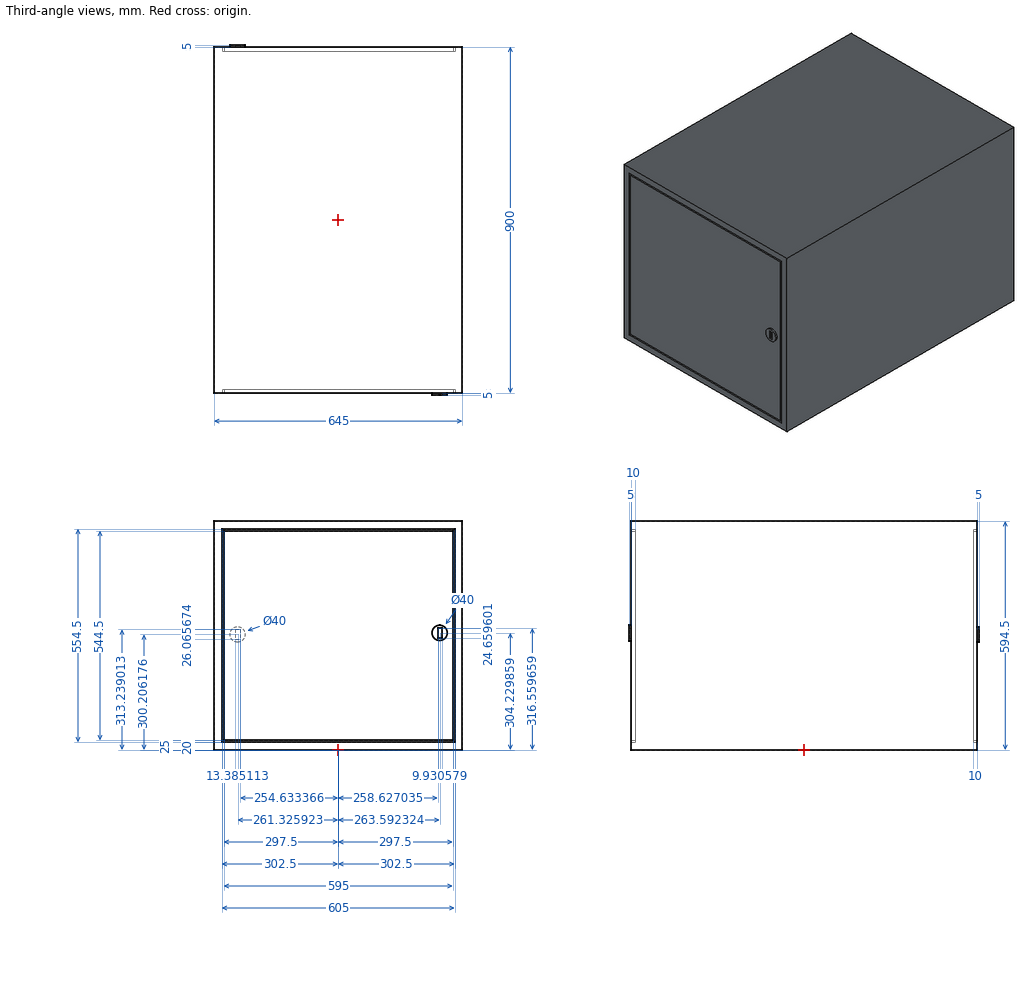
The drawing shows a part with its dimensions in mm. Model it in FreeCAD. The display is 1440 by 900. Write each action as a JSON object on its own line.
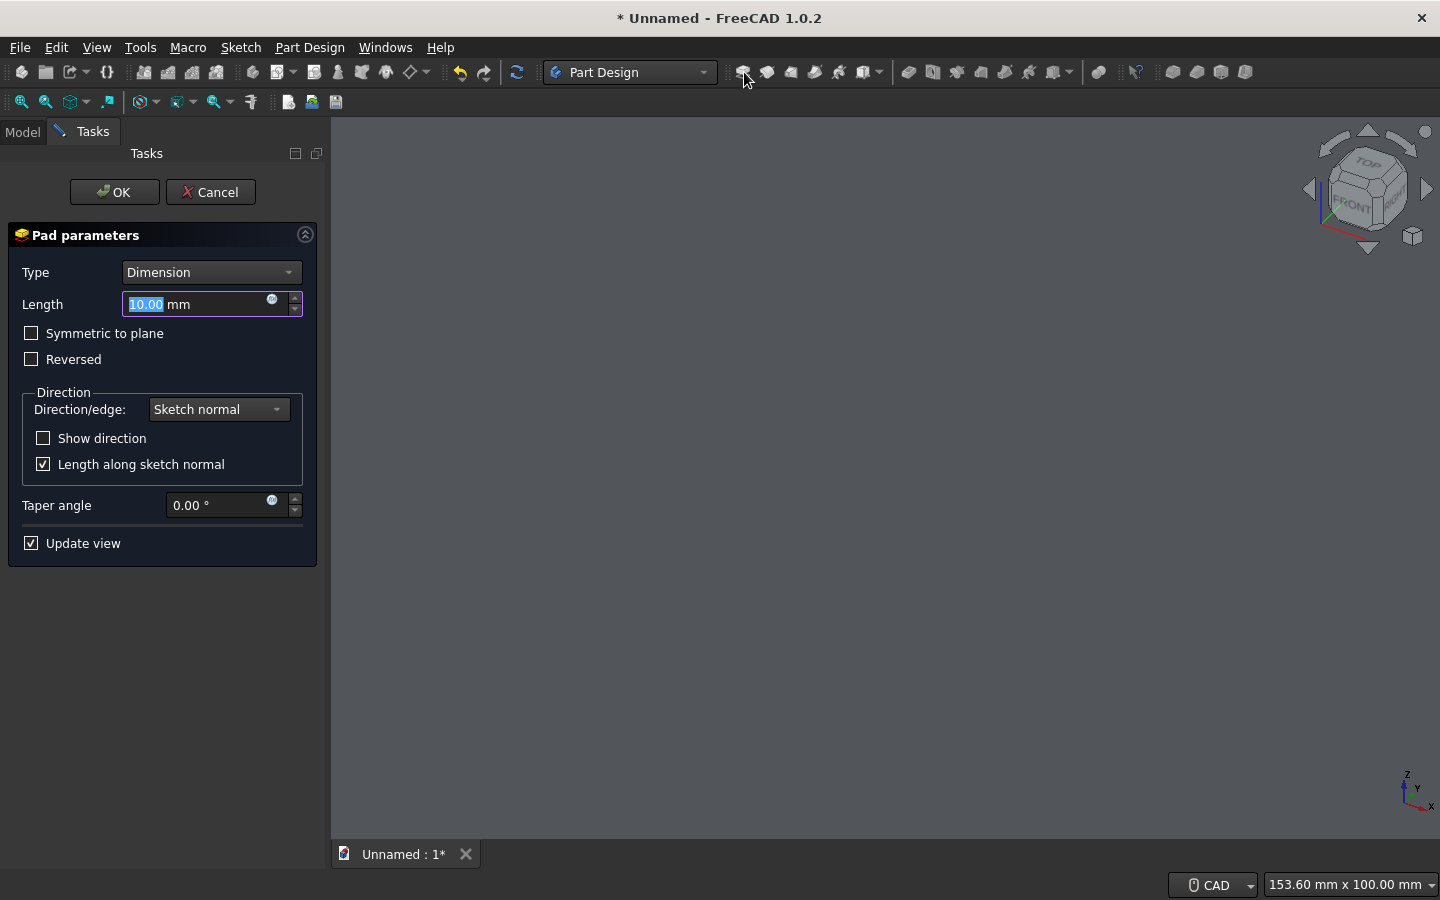
{"action": "type", "text": "594.5"}
{"action": "key", "text": "Tab"}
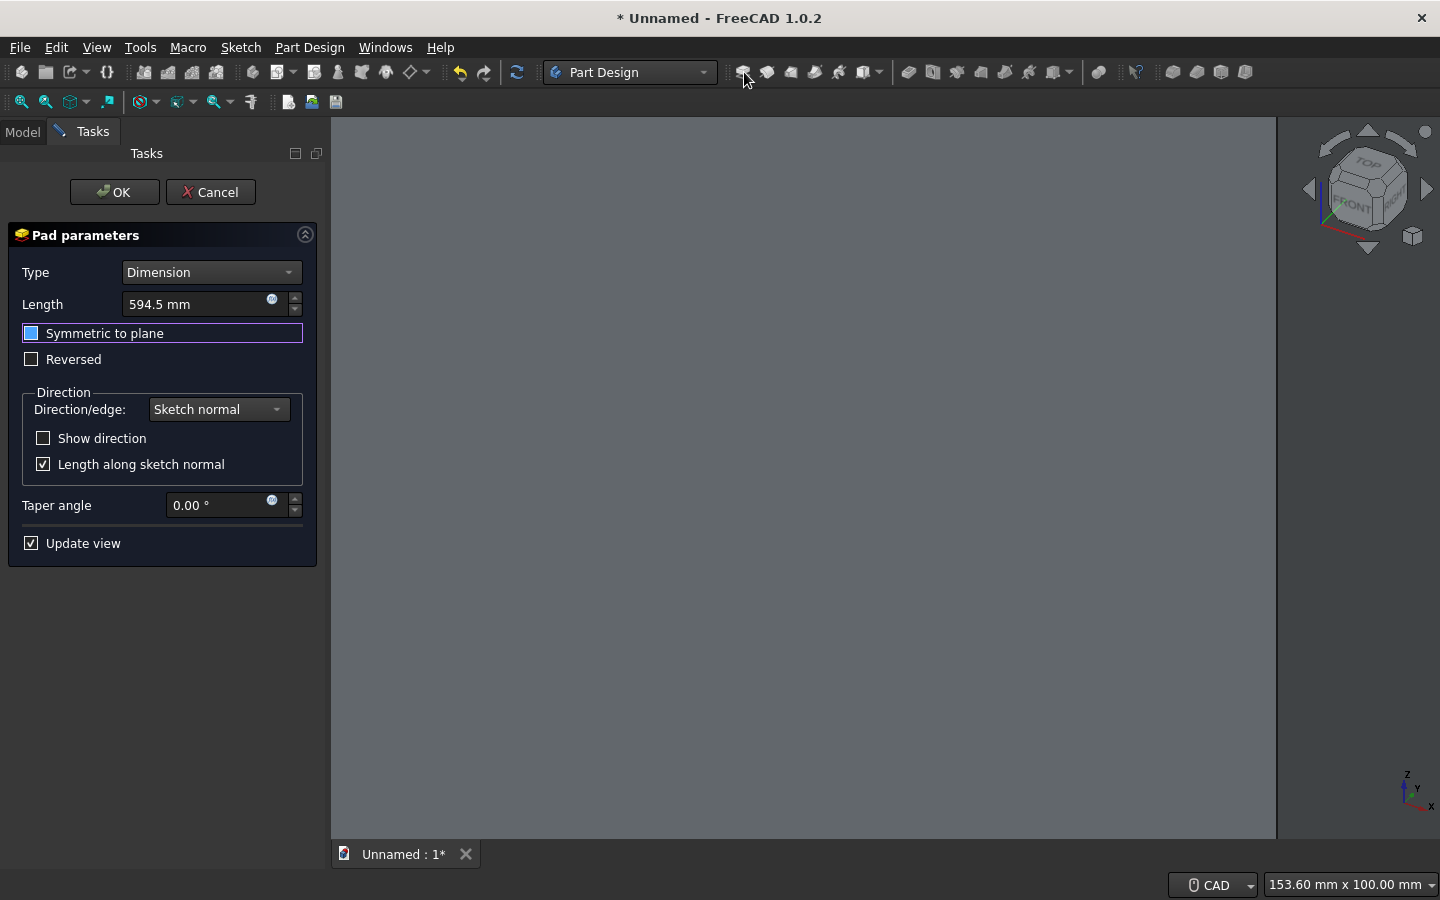
{"action": "left_click", "coordinate": [115, 192]}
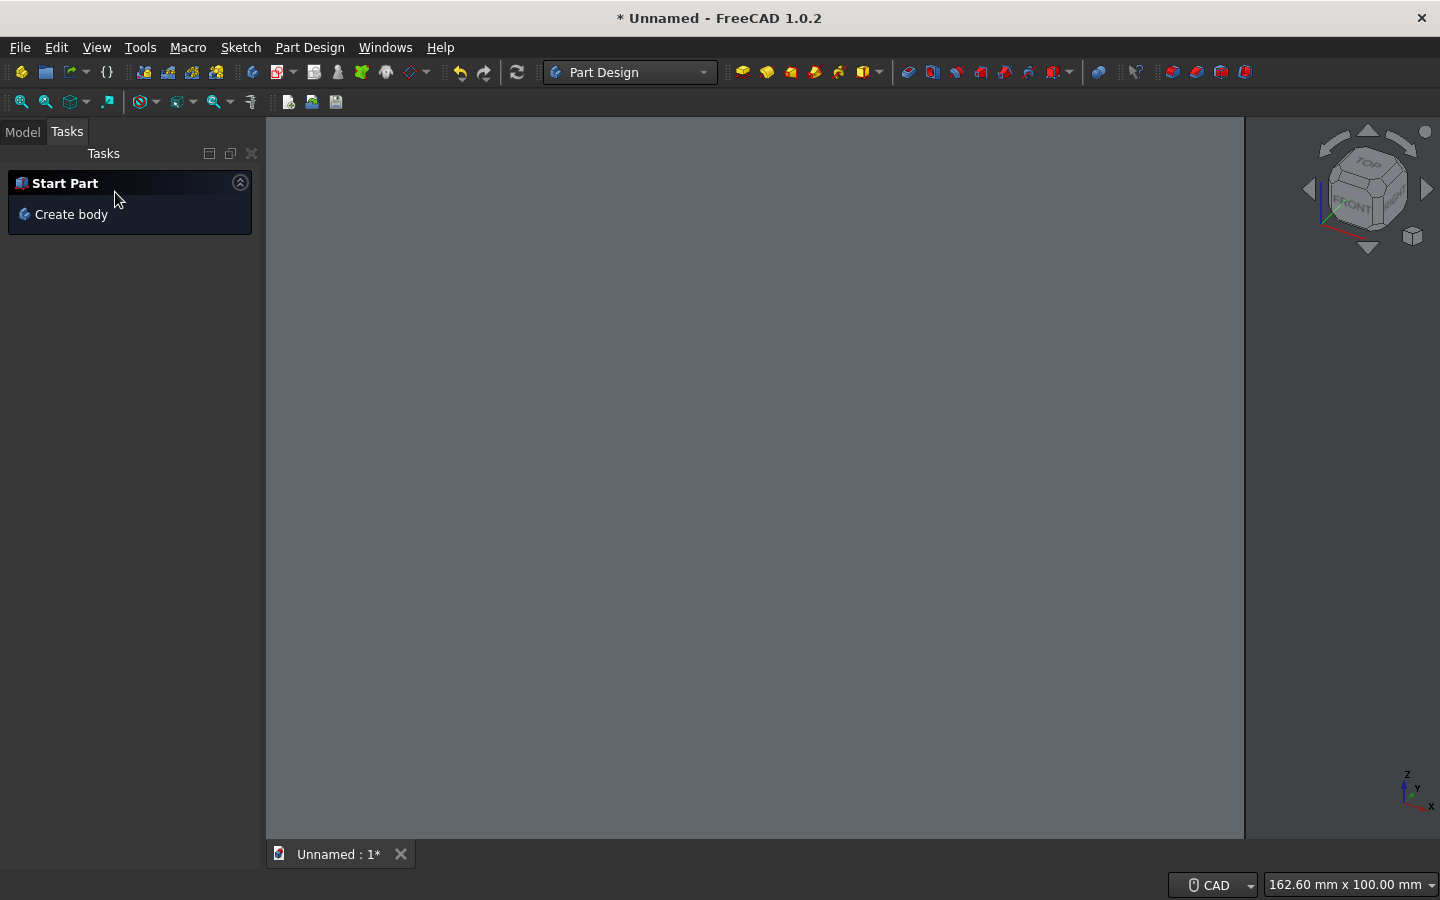
{"action": "key", "text": "v f"}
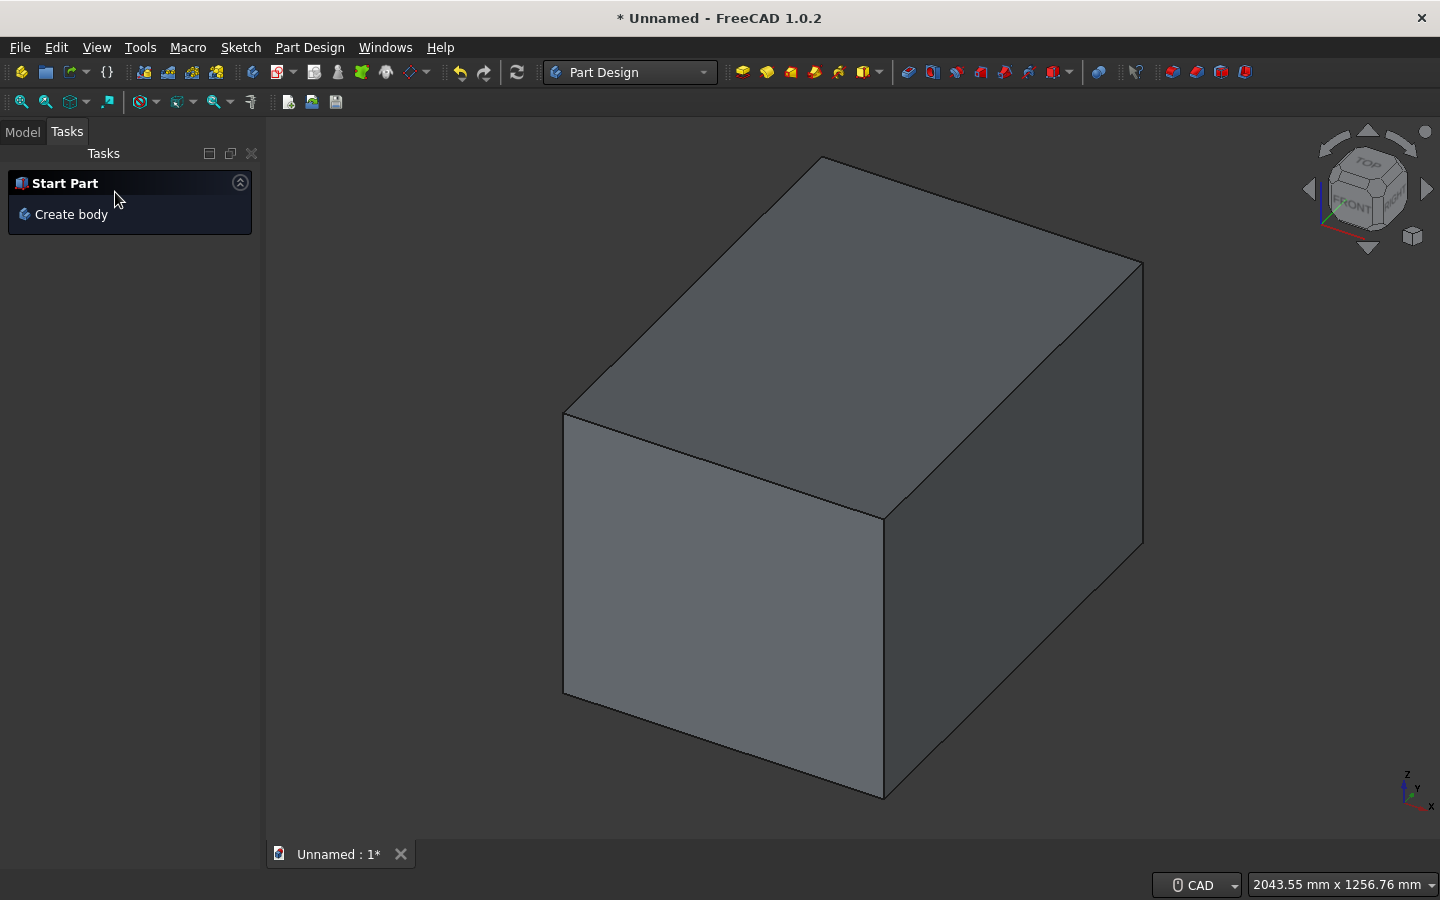
{"action": "left_click", "coordinate": [724, 605]}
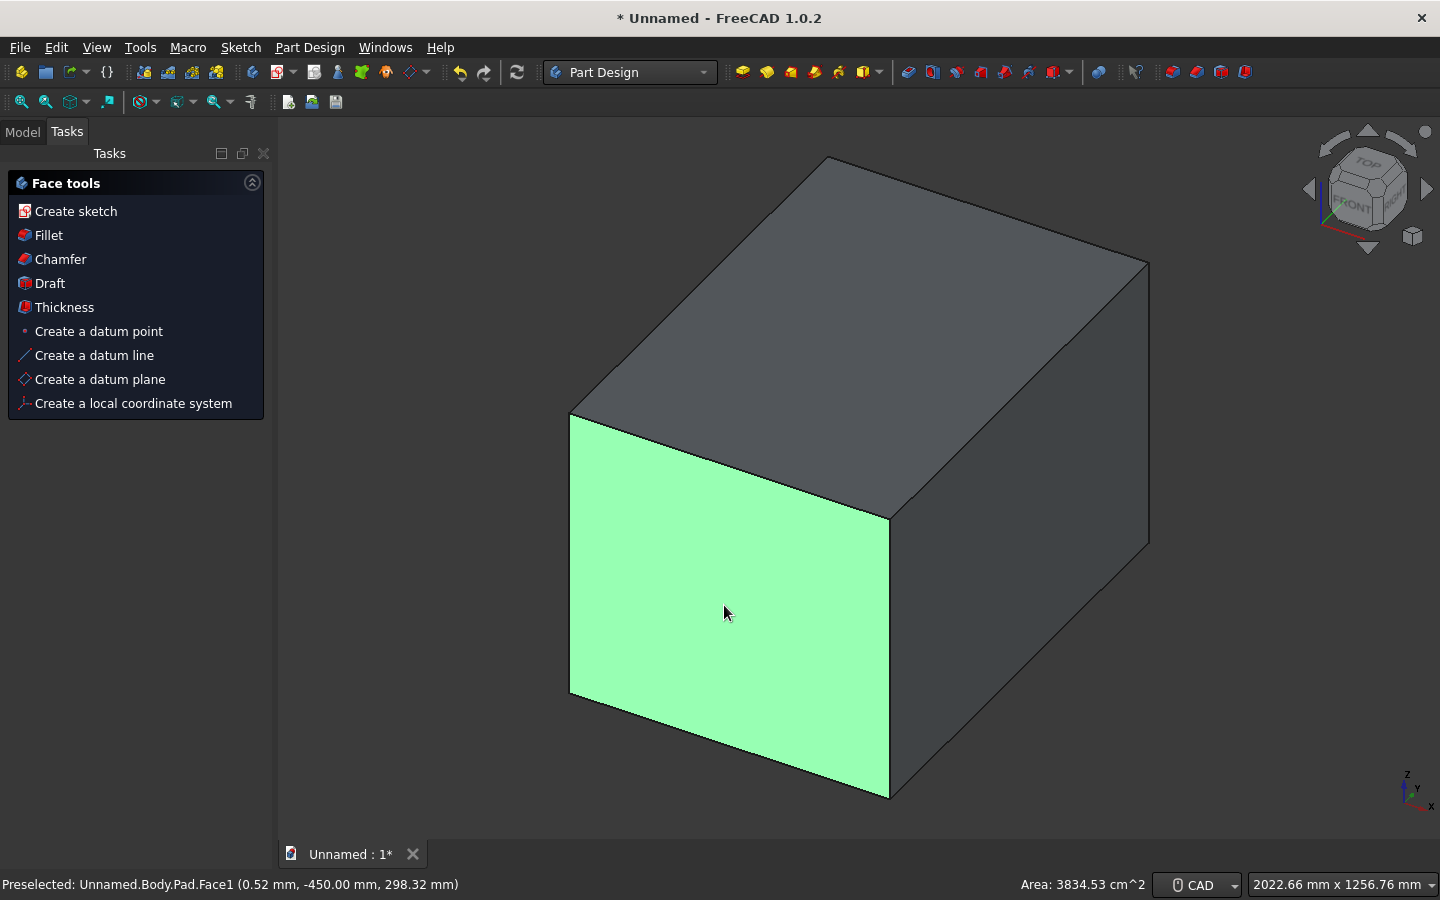
{"action": "left_click", "coordinate": [278, 72]}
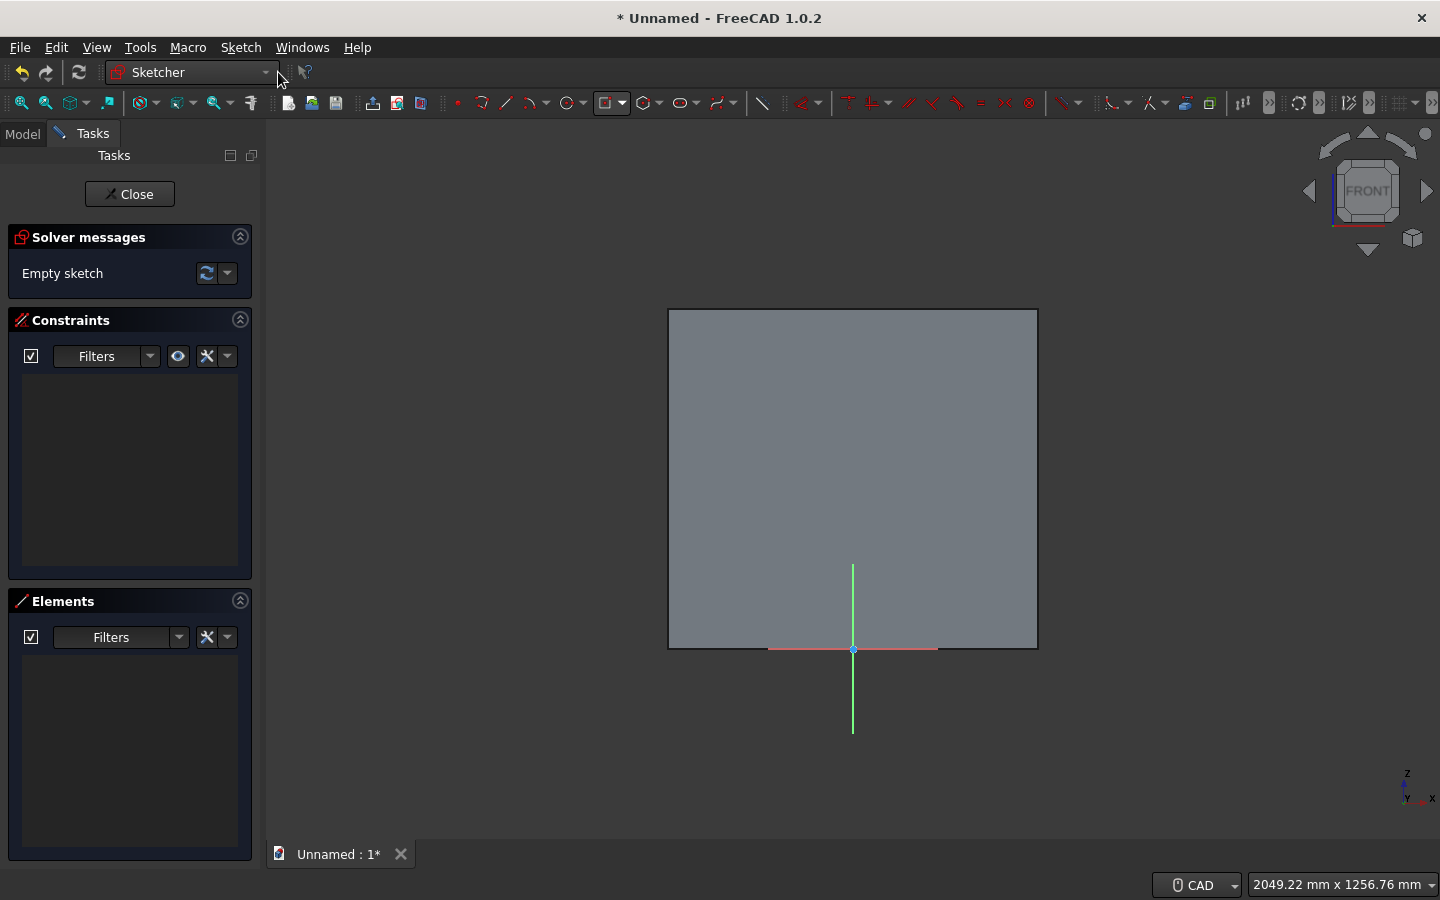
{"action": "scroll", "coordinate": [992, 496], "scroll_direction": "up", "scroll_amount": 2}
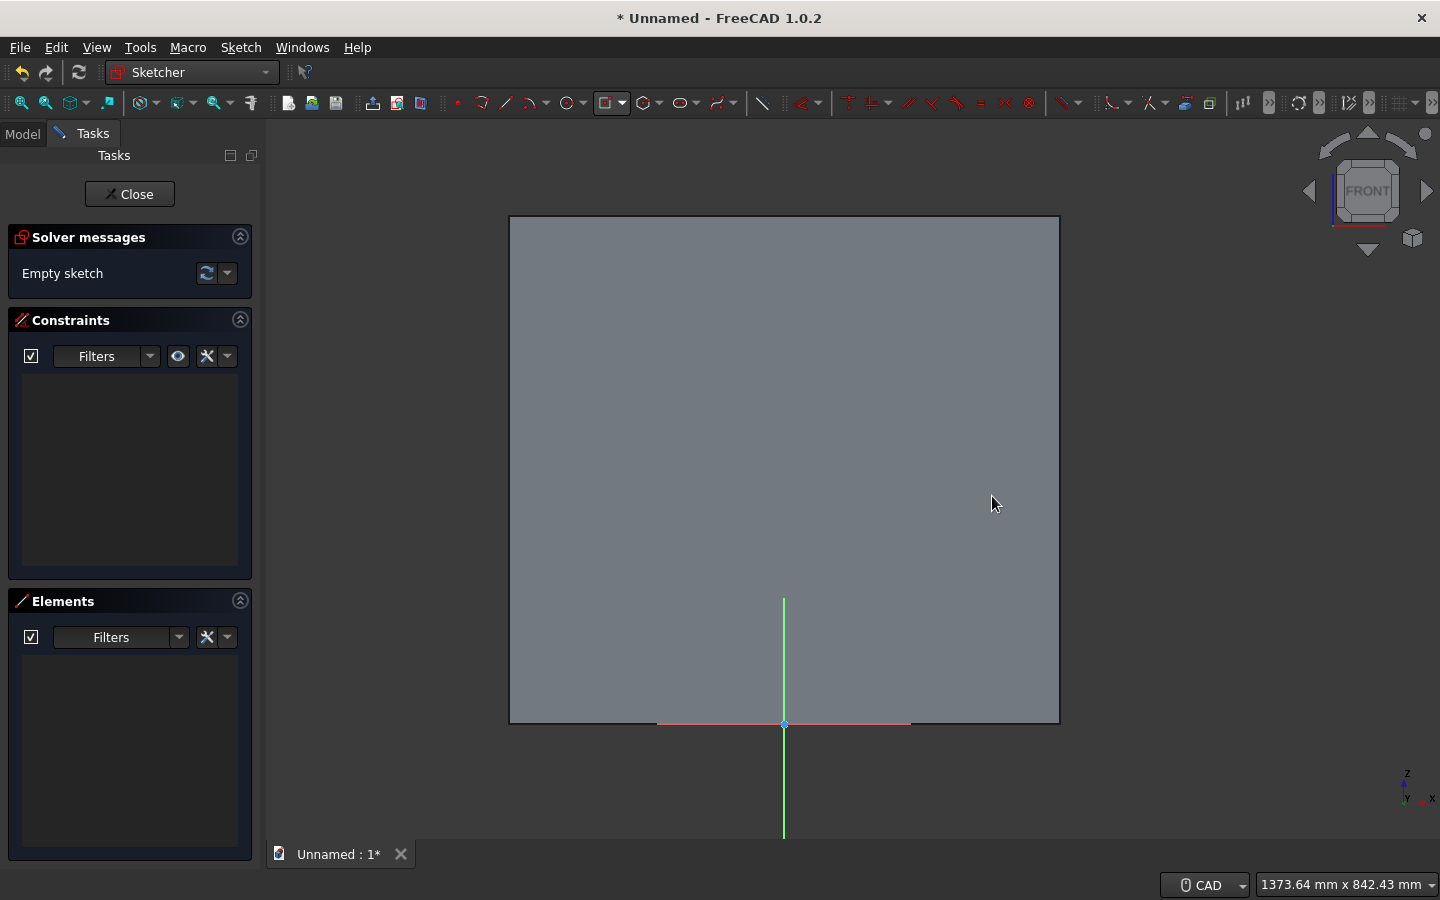
{"action": "key", "text": "g r"}